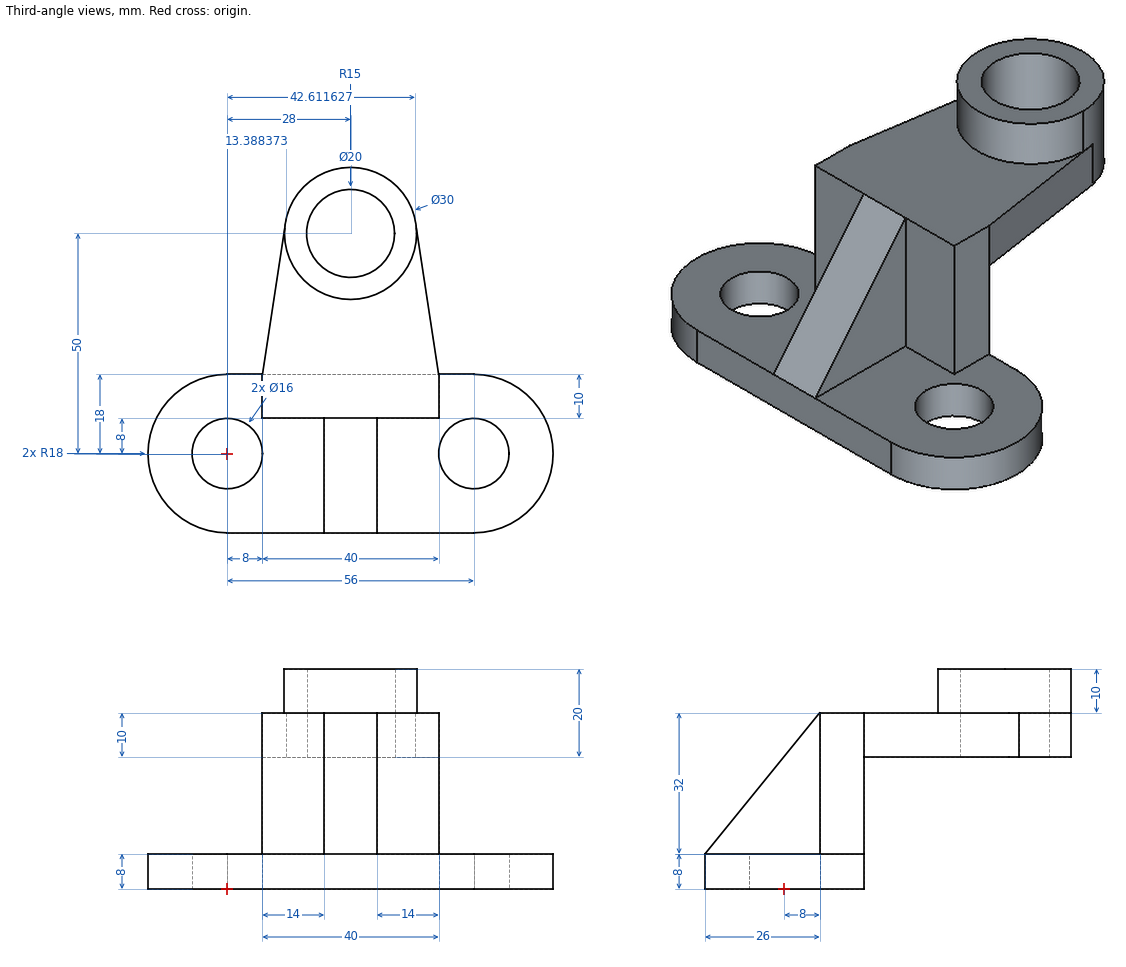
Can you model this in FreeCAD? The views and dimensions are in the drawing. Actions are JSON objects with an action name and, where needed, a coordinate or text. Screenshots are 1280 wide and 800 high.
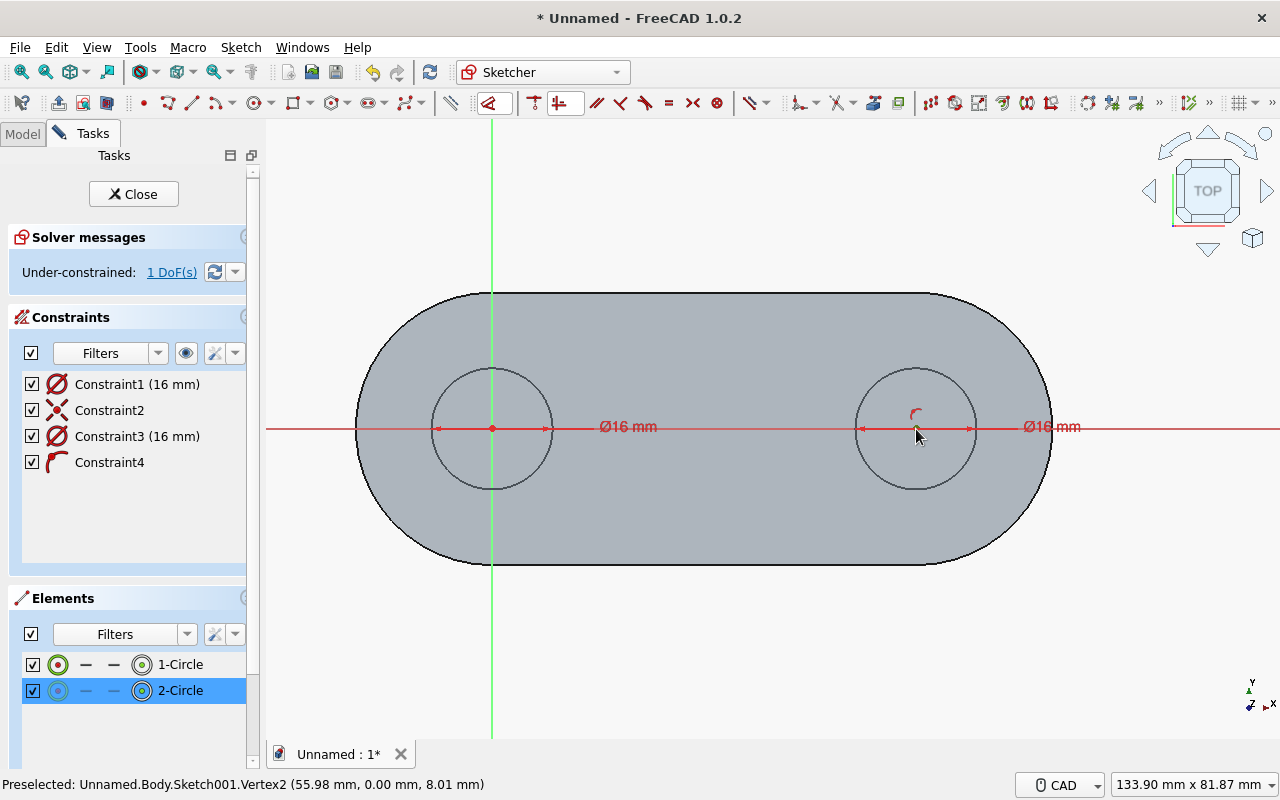
{"action": "left_click", "coordinate": [506, 104]}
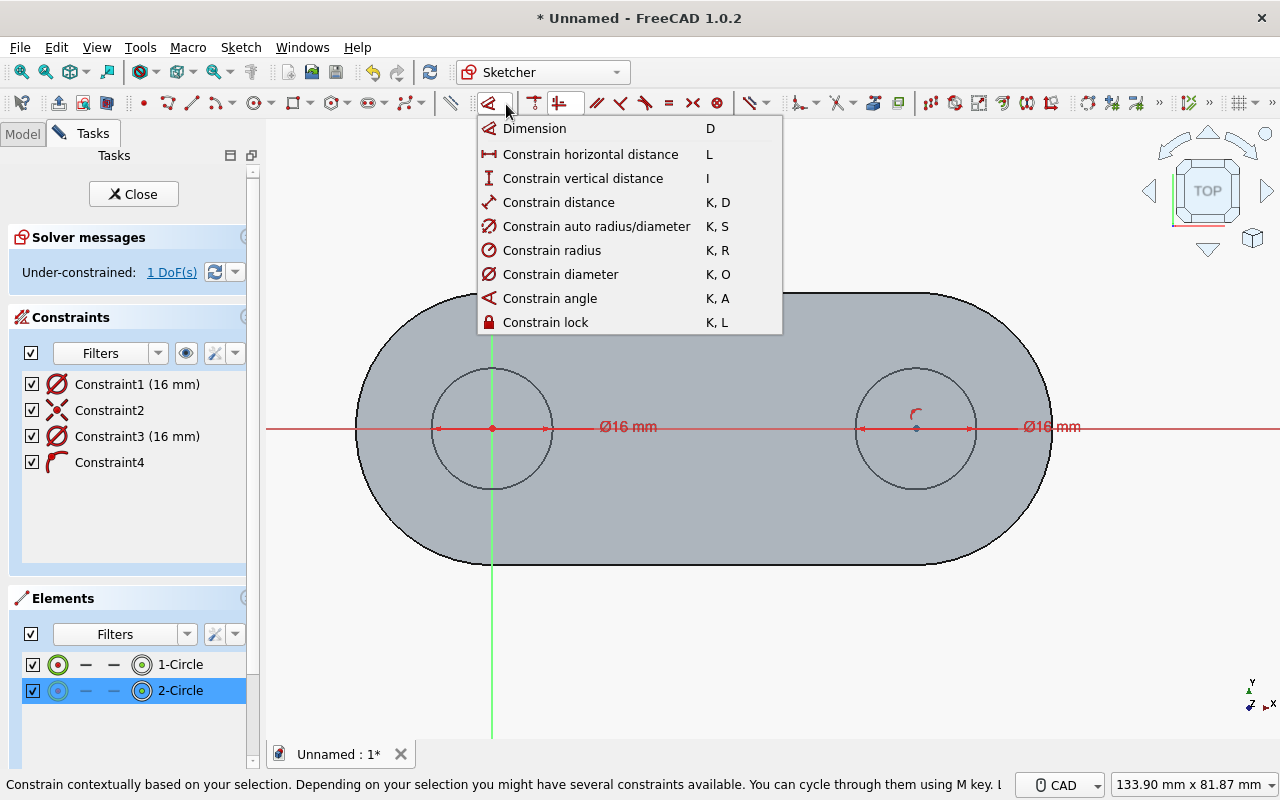
{"action": "left_click", "coordinate": [630, 154]}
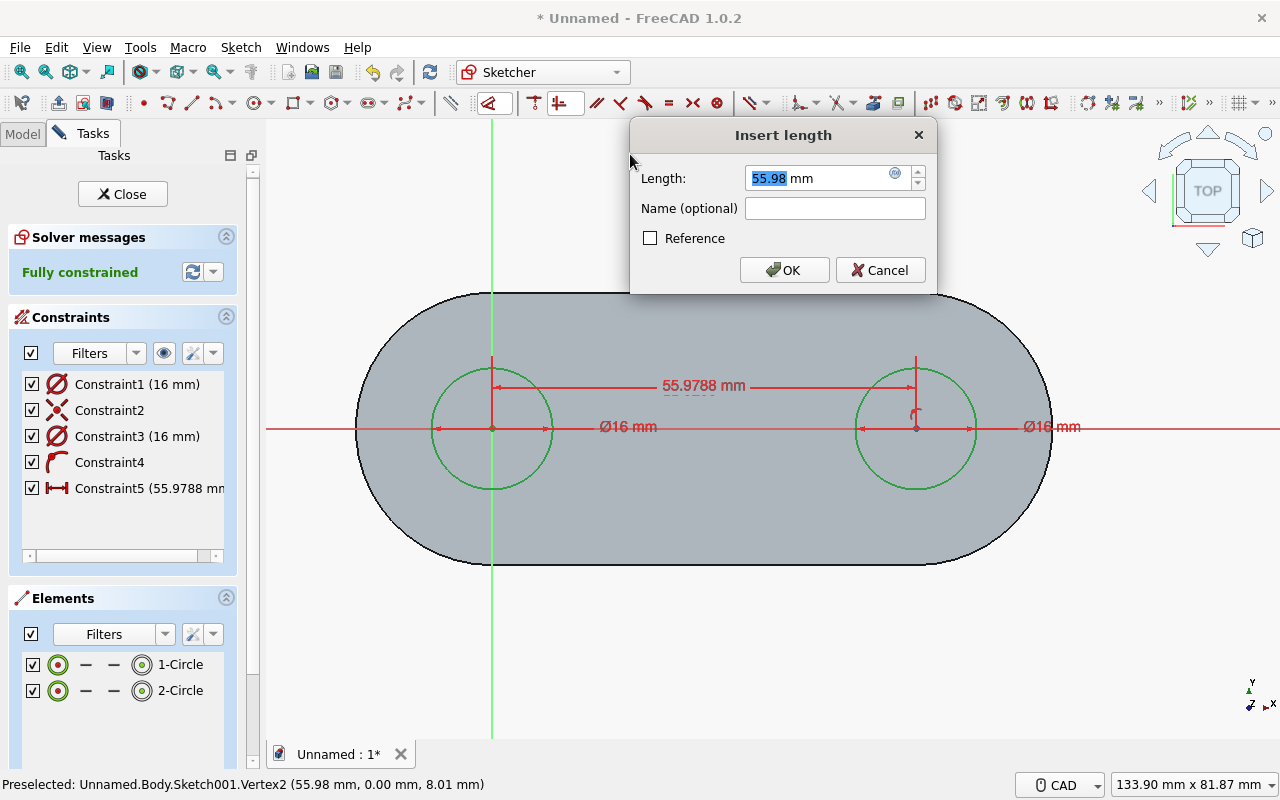
{"action": "type", "text": "56"}
{"action": "key", "text": "Return"}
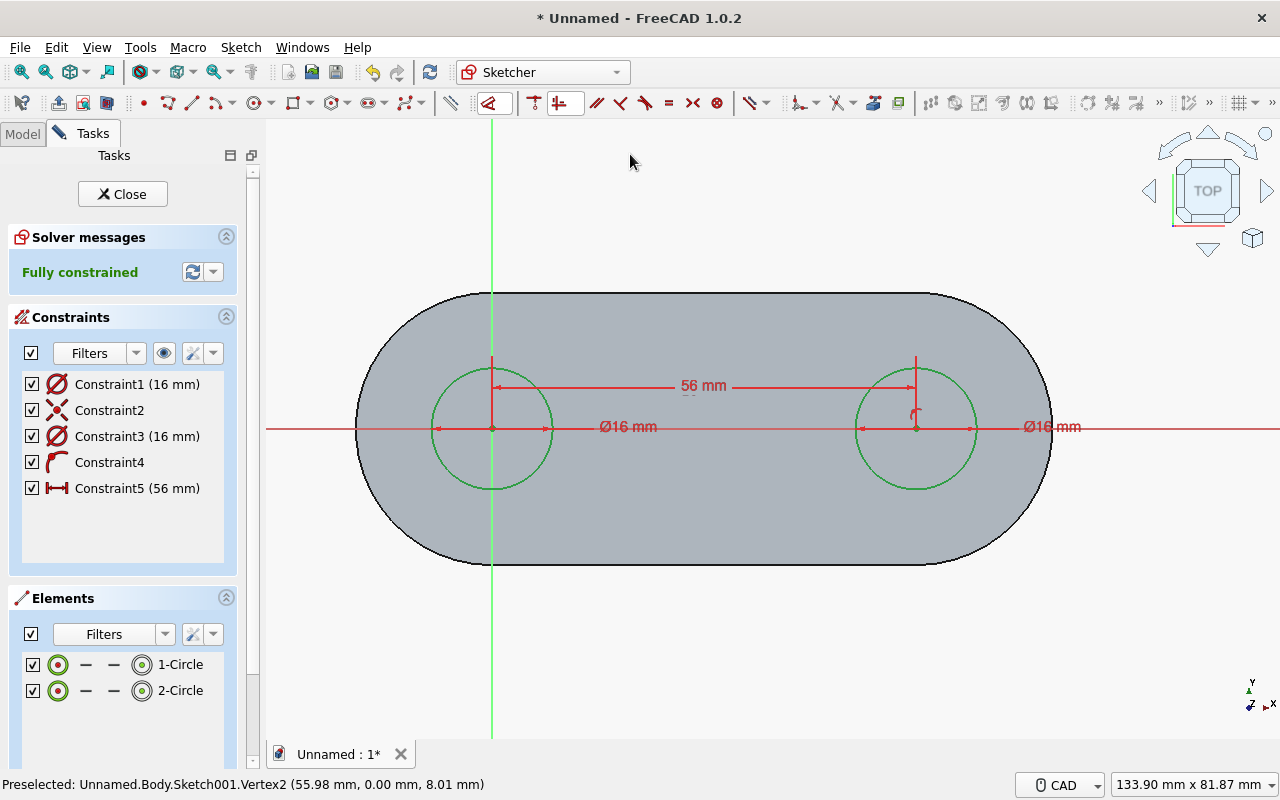
{"action": "left_click", "coordinate": [123, 194]}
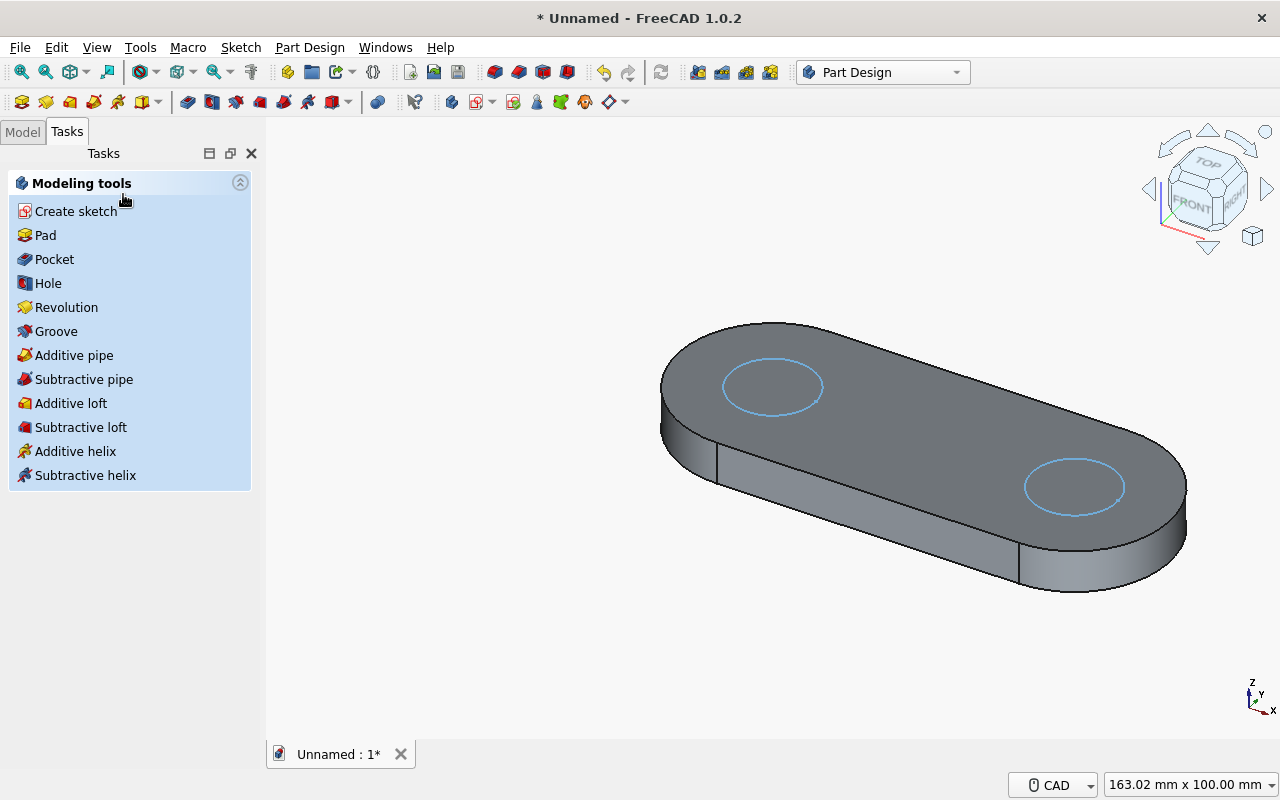
{"action": "left_click", "coordinate": [188, 102]}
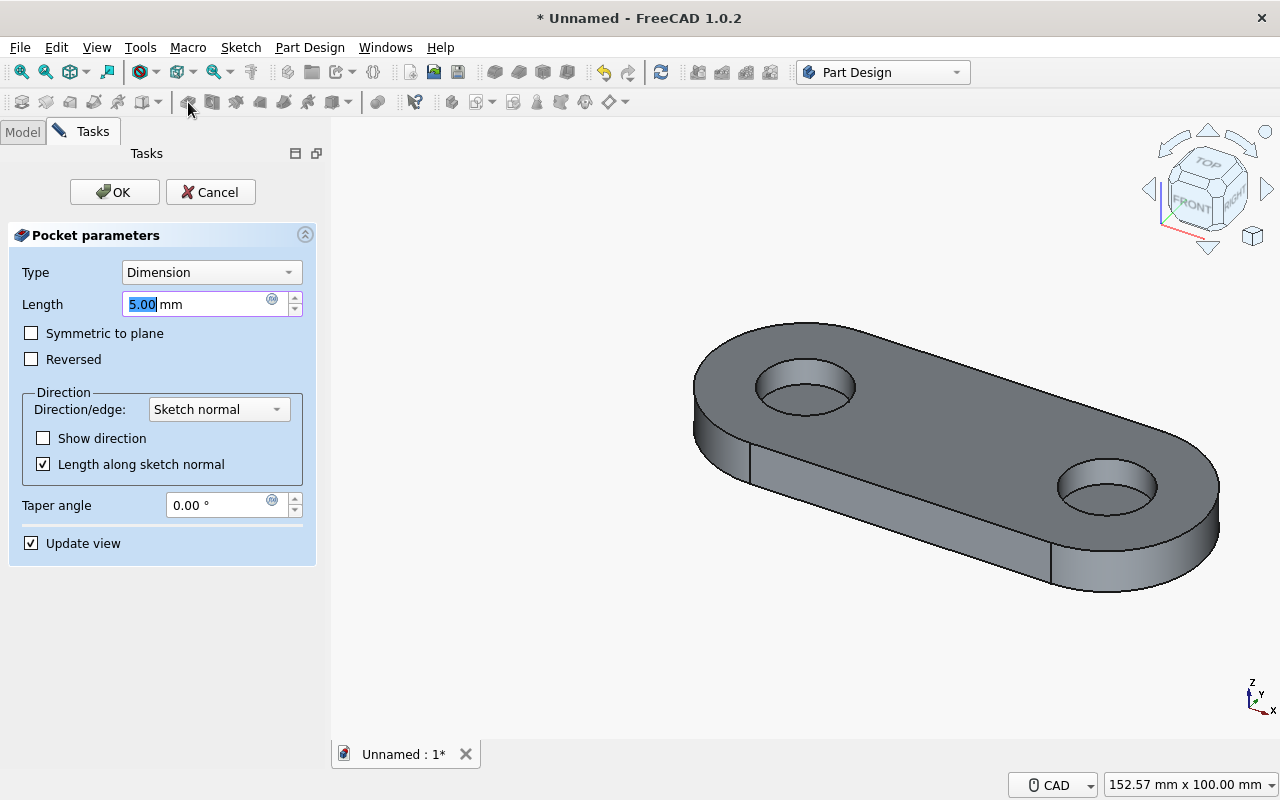
{"action": "type", "text": "8"}
{"action": "key", "text": "Tab"}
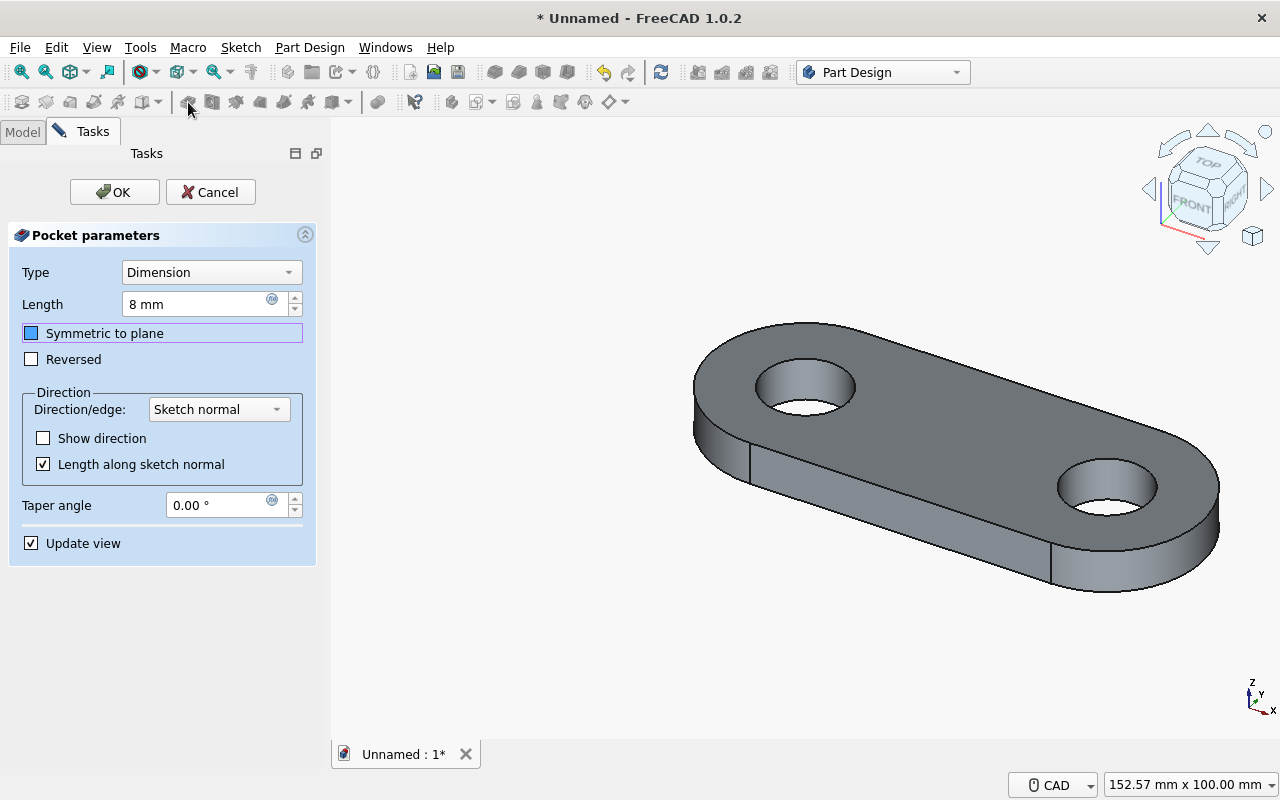
{"action": "left_click", "coordinate": [115, 192]}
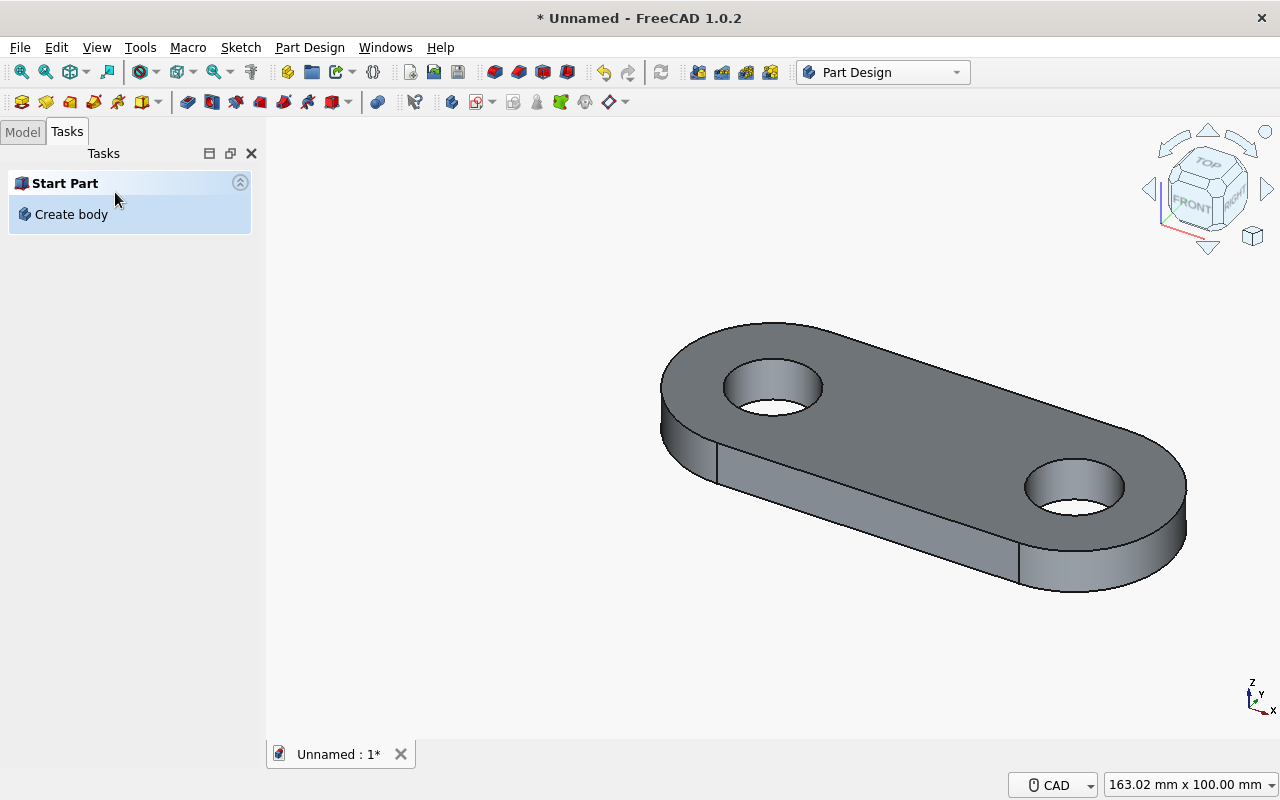
{"action": "left_click", "coordinate": [924, 436]}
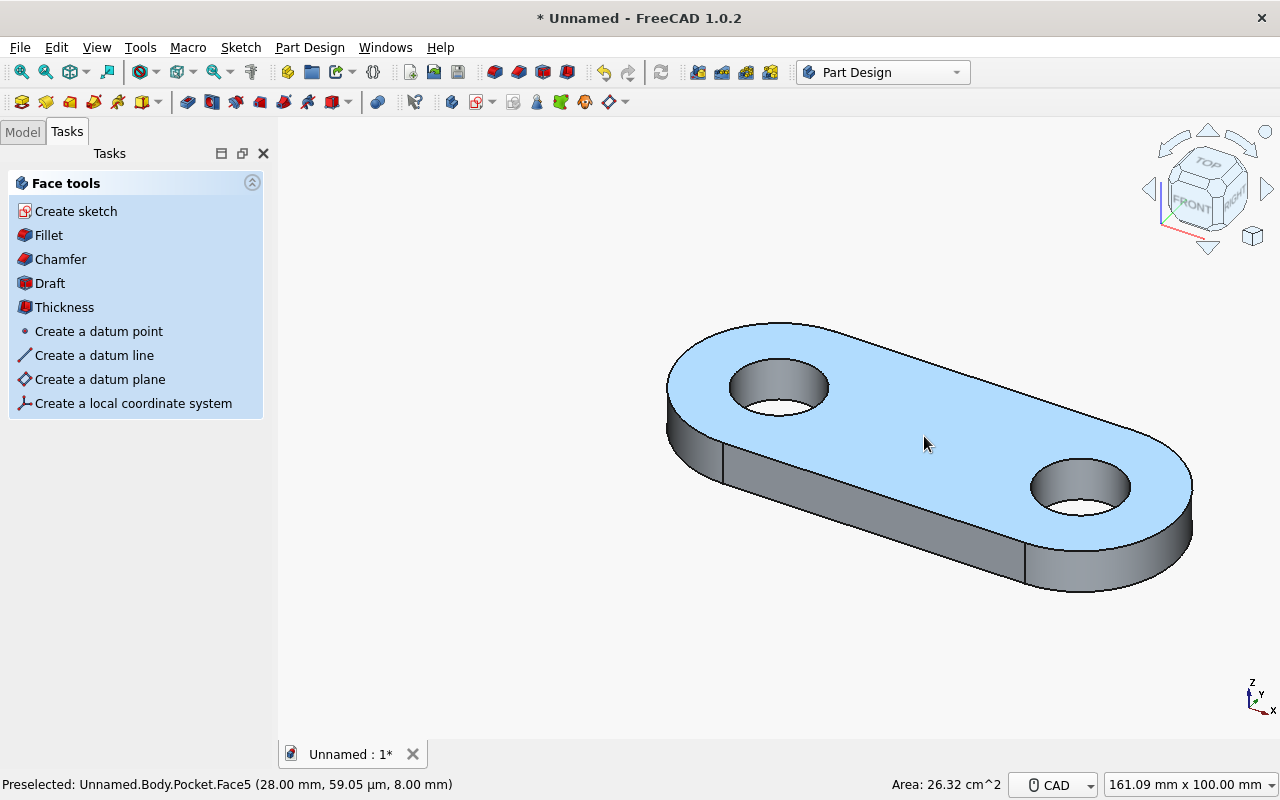
{"action": "left_click", "coordinate": [476, 102]}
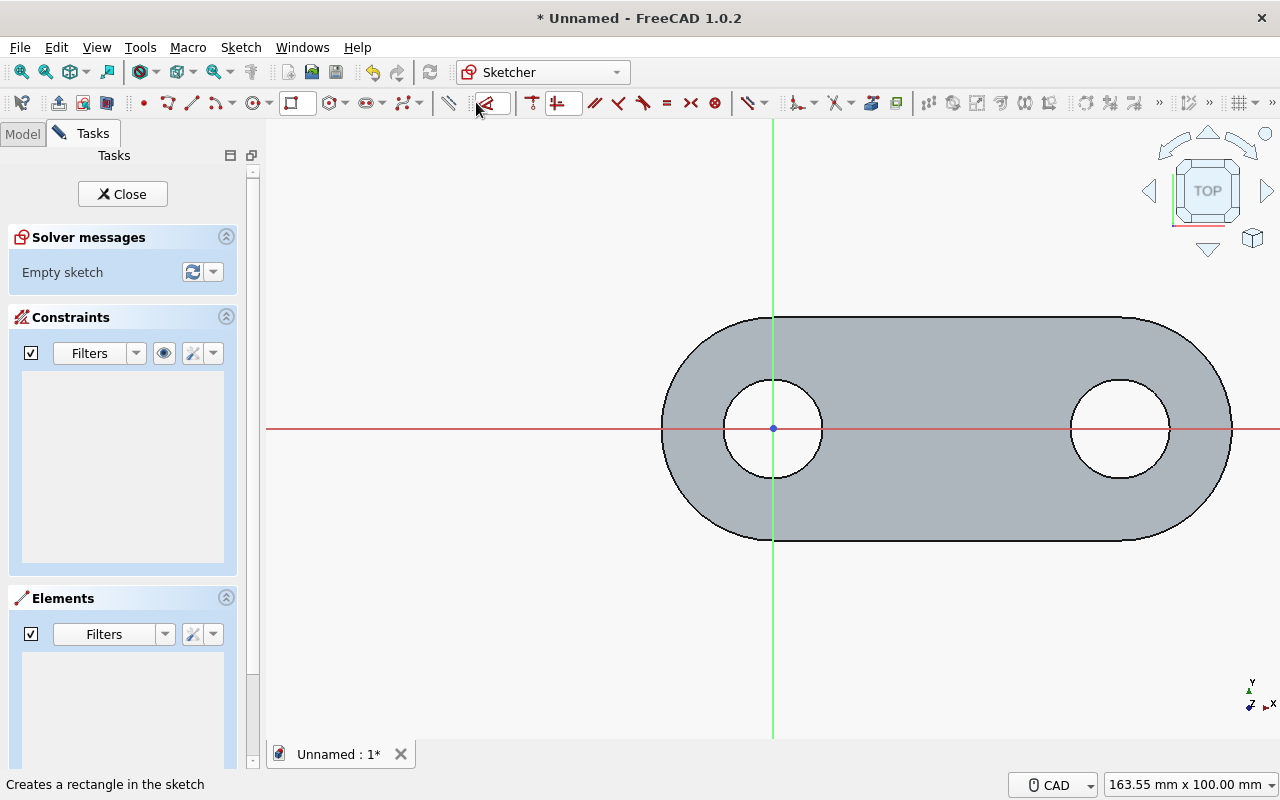
{"action": "scroll", "coordinate": [1115, 305], "scroll_direction": "up", "scroll_amount": 3}